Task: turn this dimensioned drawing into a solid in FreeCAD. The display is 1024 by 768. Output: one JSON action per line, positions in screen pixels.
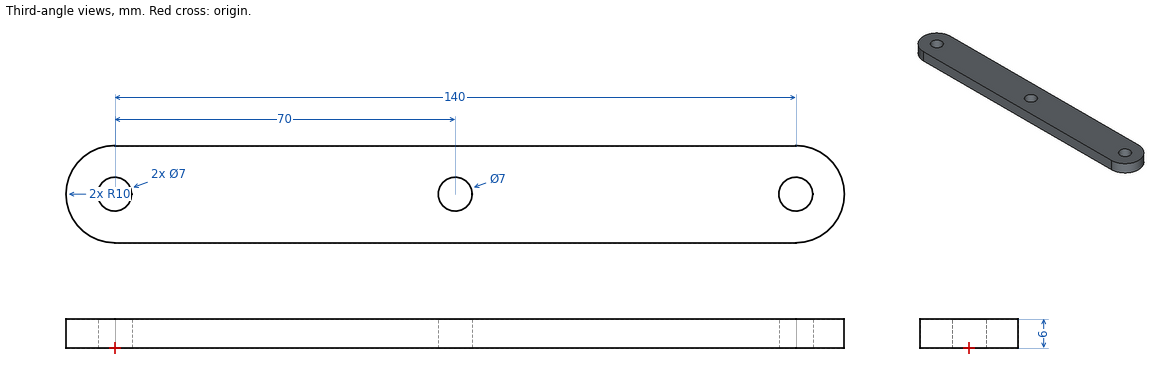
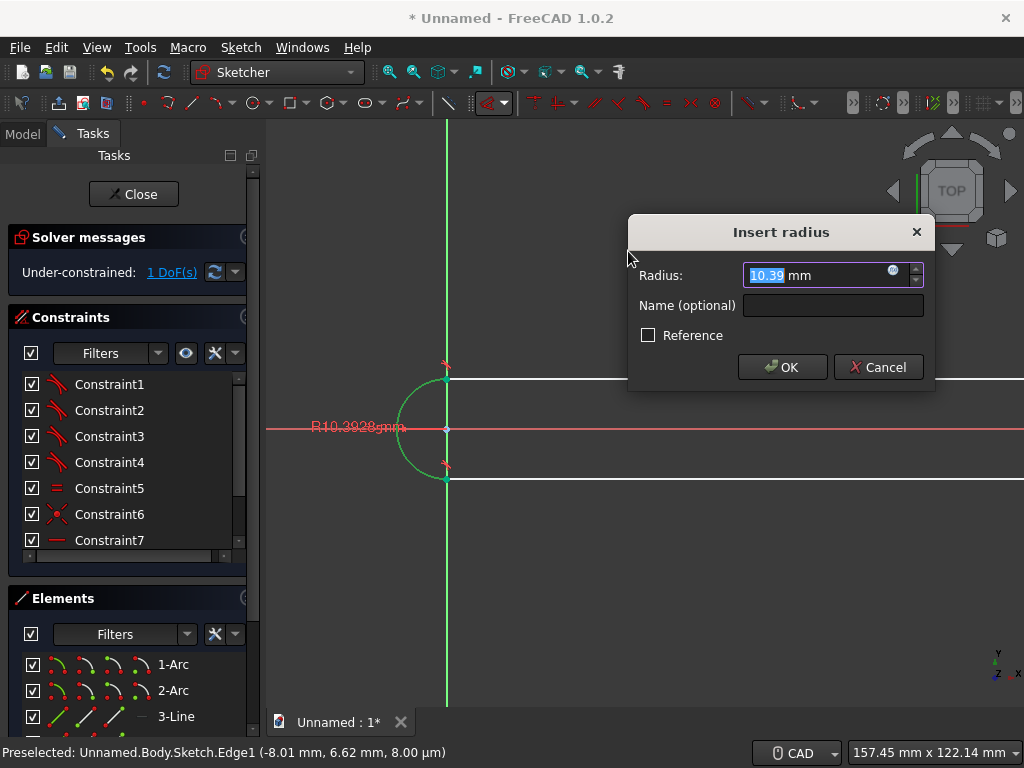
{"action": "type", "text": "10"}
{"action": "key", "text": "Return"}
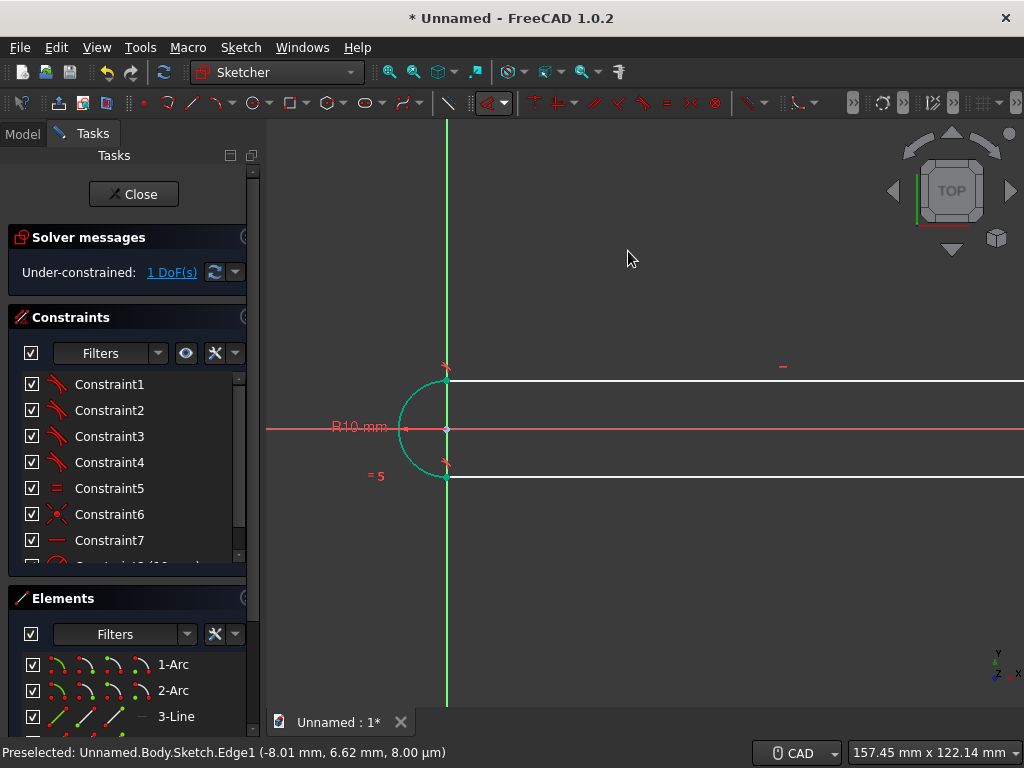
{"action": "left_click", "coordinate": [649, 381]}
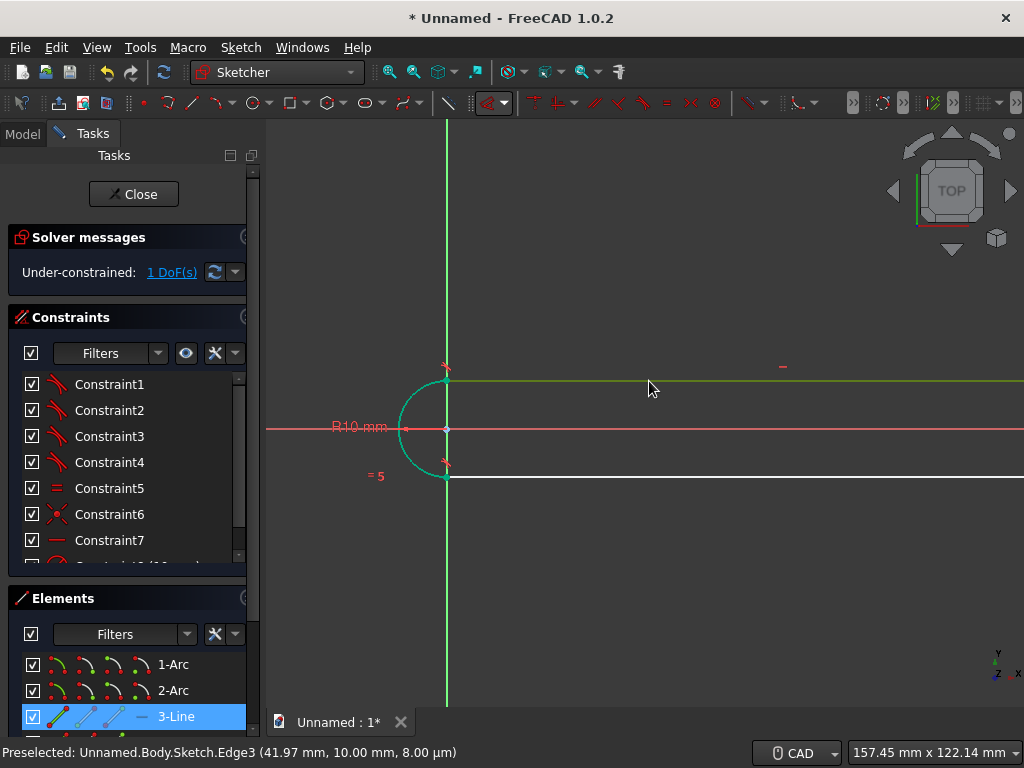
{"action": "key", "text": "l"}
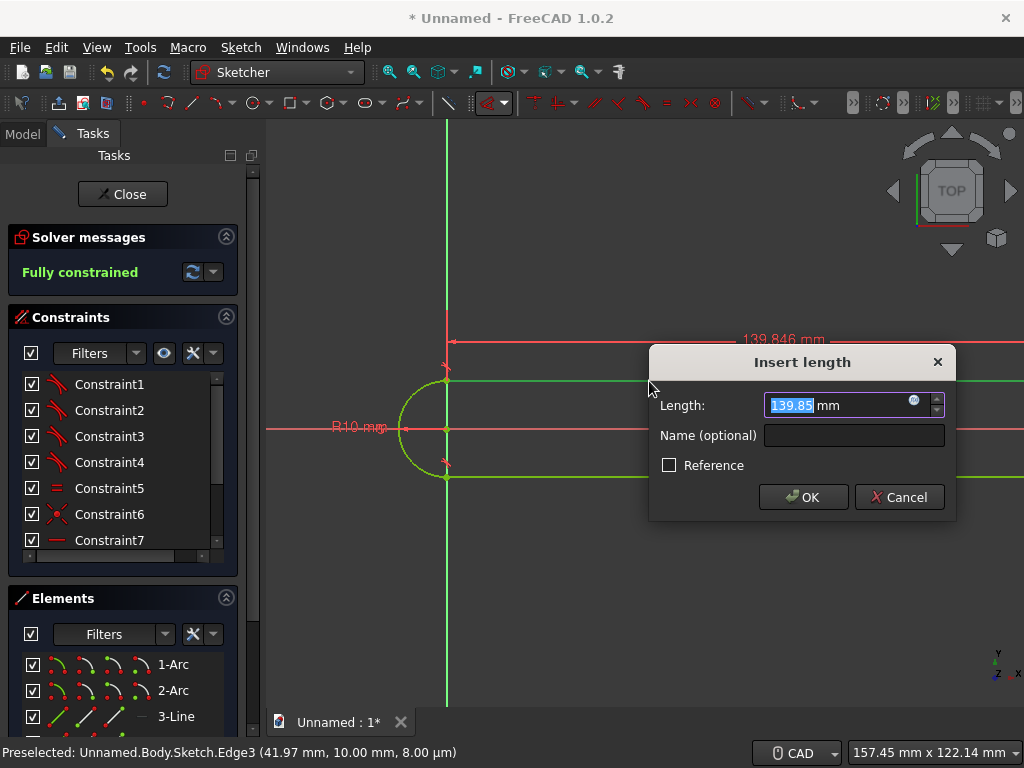
{"action": "type", "text": "140"}
{"action": "key", "text": "Return"}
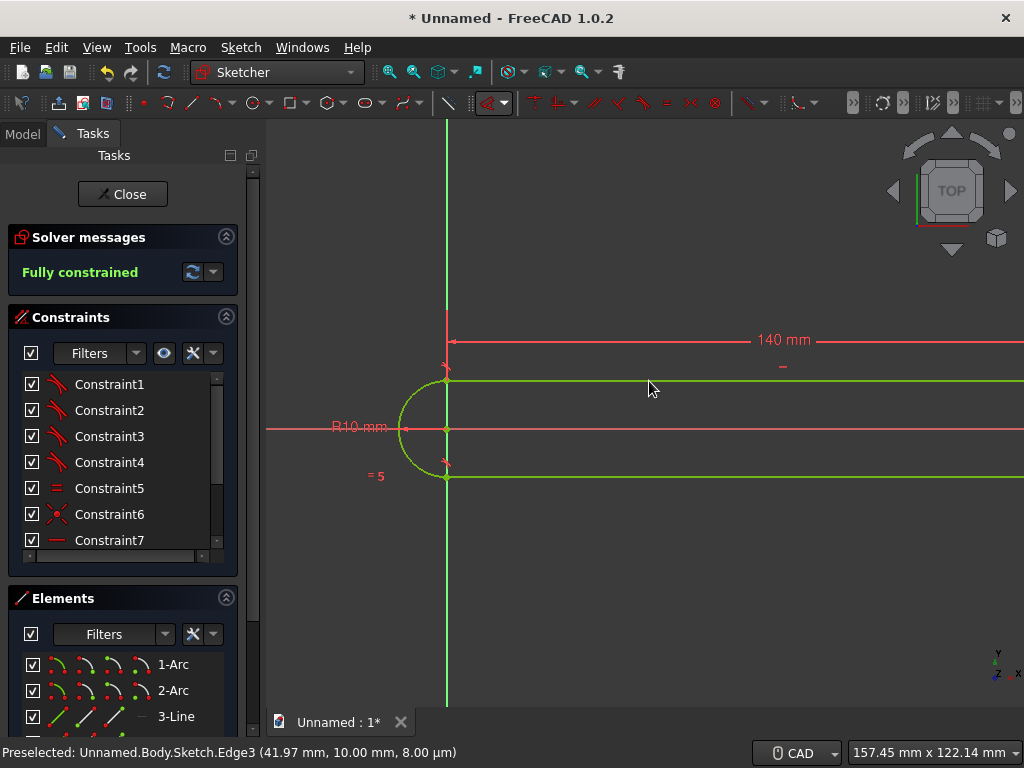
{"action": "left_click", "coordinate": [123, 194]}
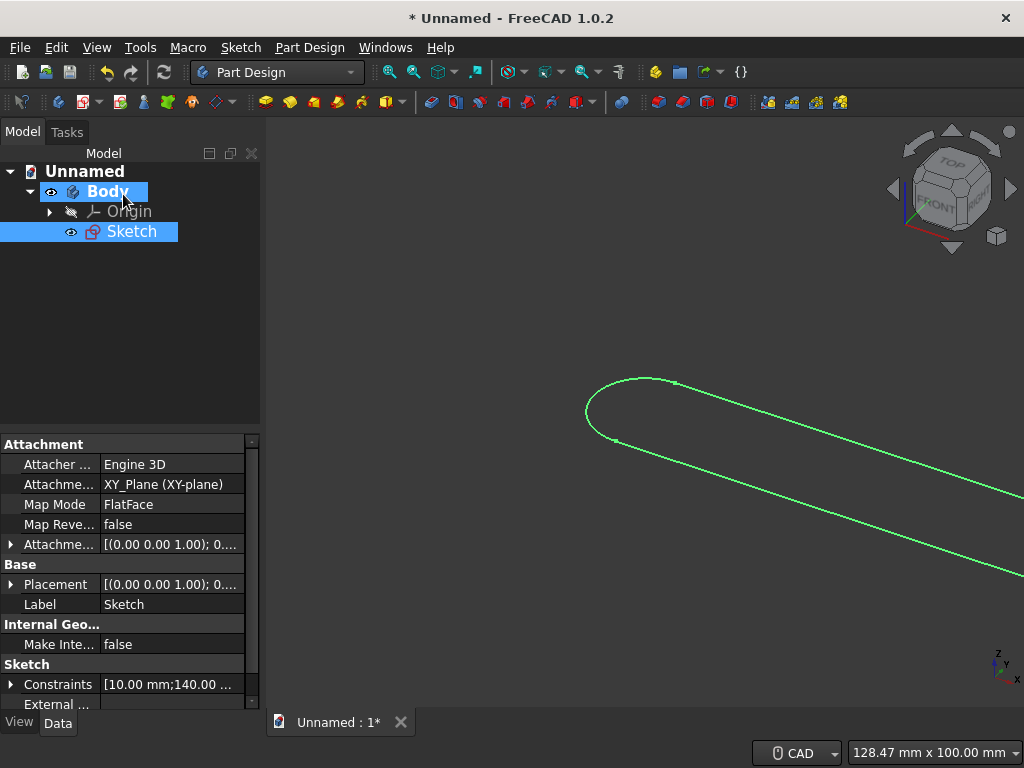
{"action": "left_click", "coordinate": [266, 102]}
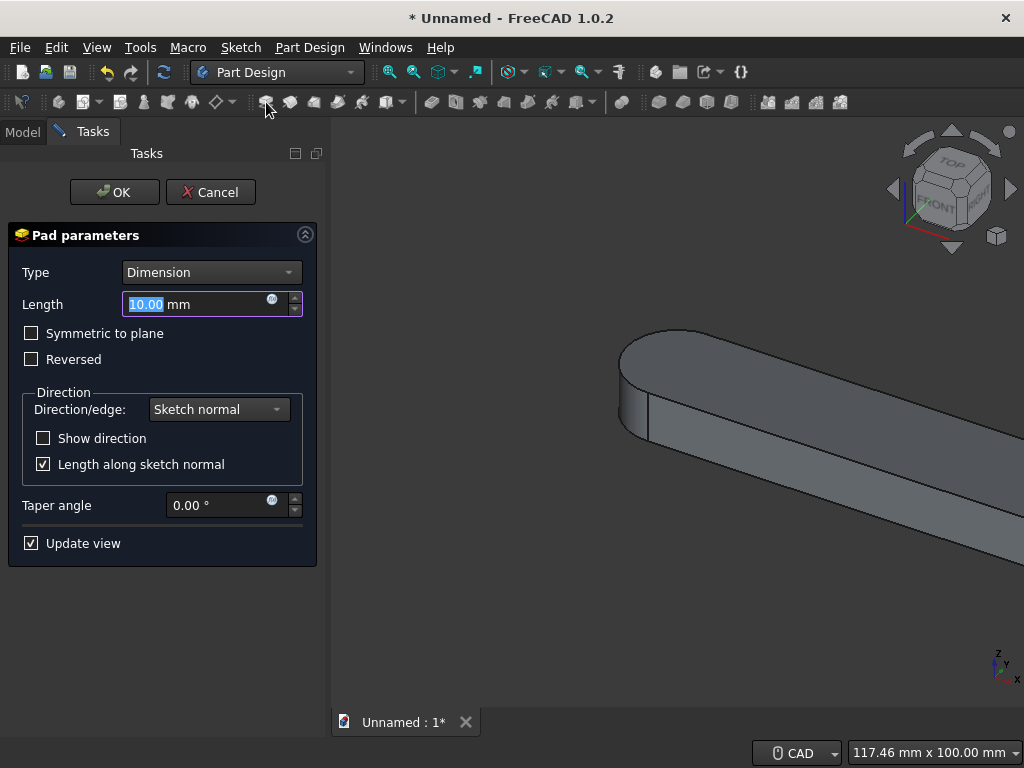
{"action": "type", "text": "6"}
{"action": "key", "text": "Tab"}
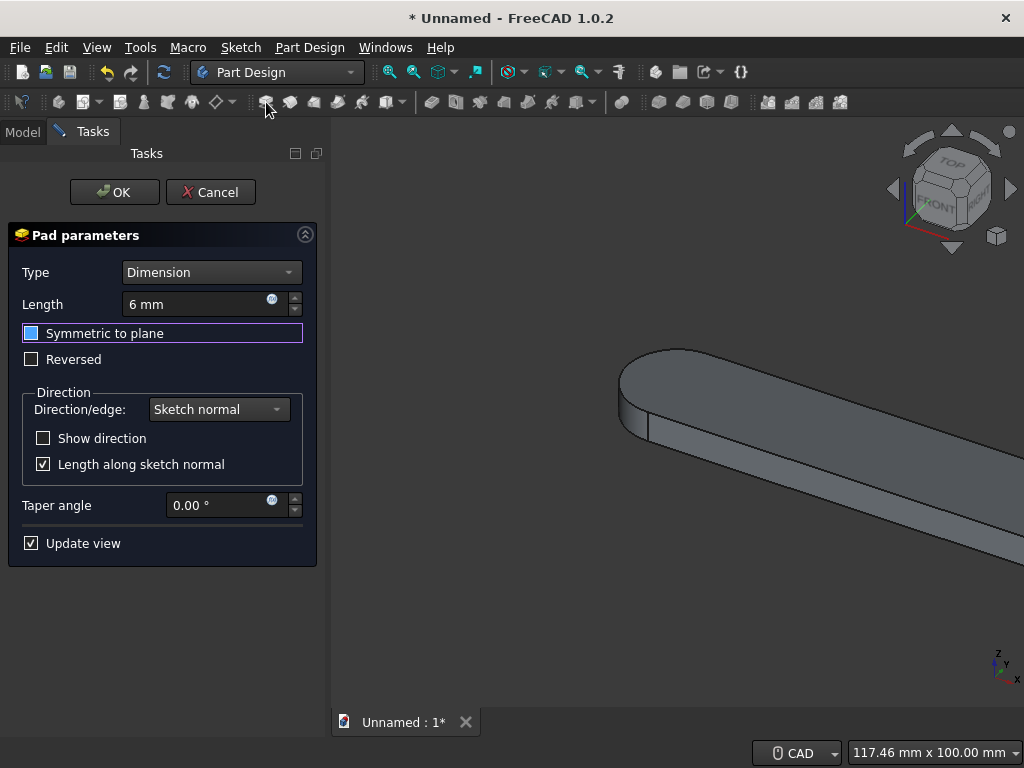
{"action": "left_click", "coordinate": [115, 192]}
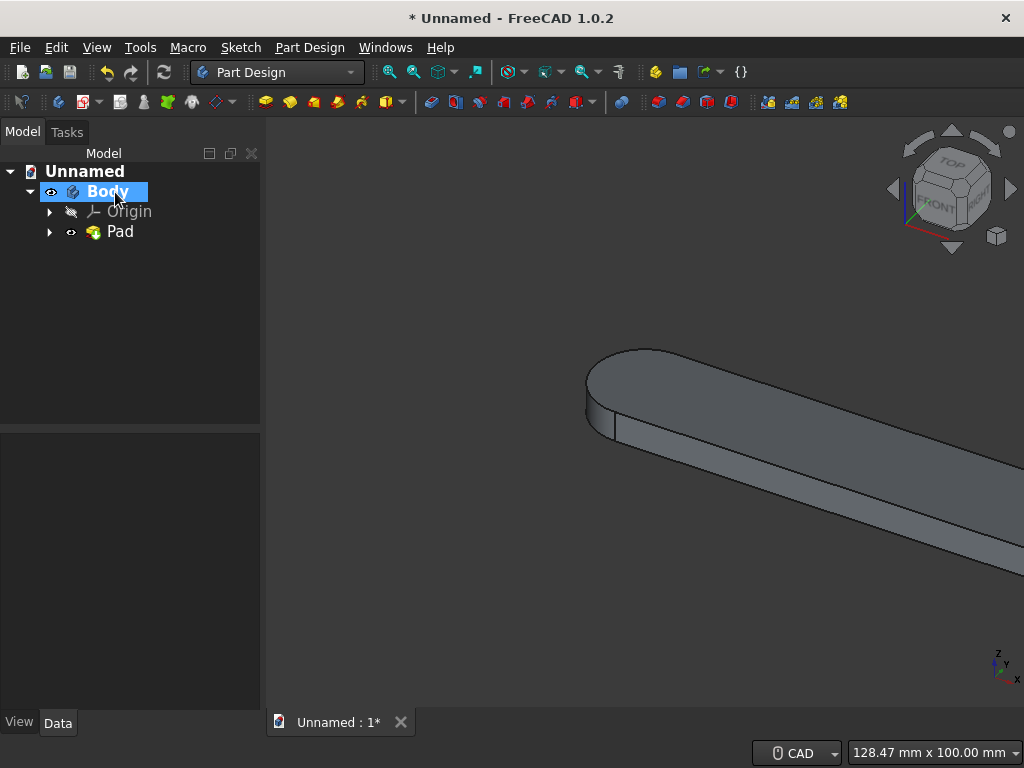
{"action": "left_click", "coordinate": [390, 72]}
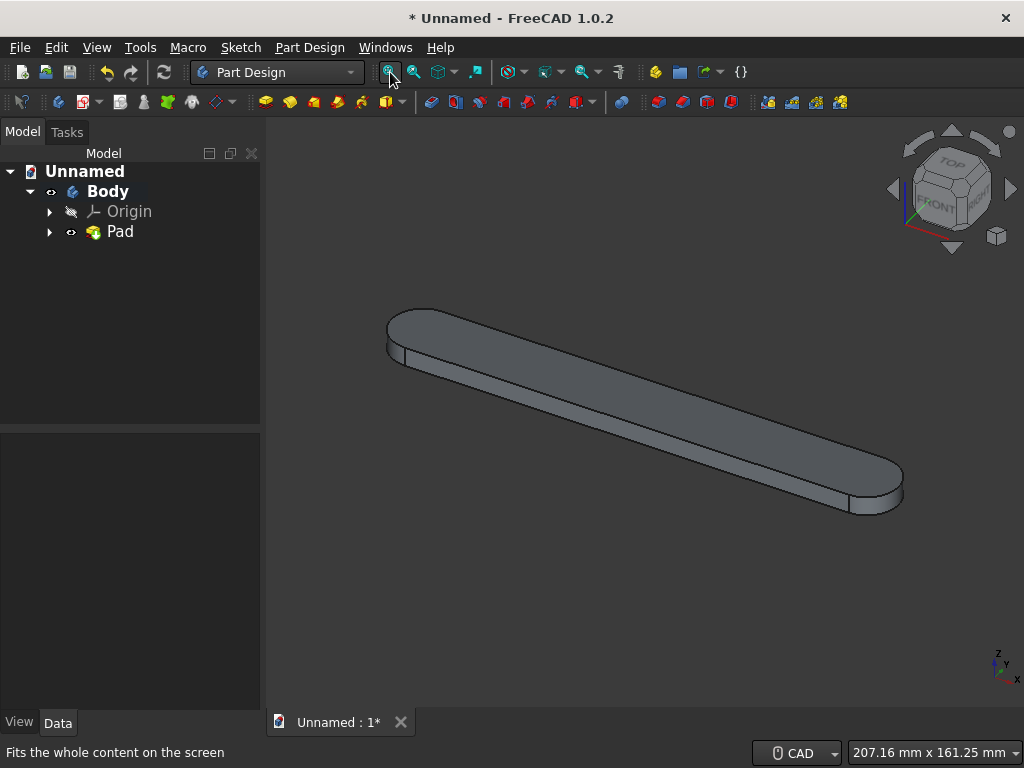
{"action": "left_click", "coordinate": [862, 474]}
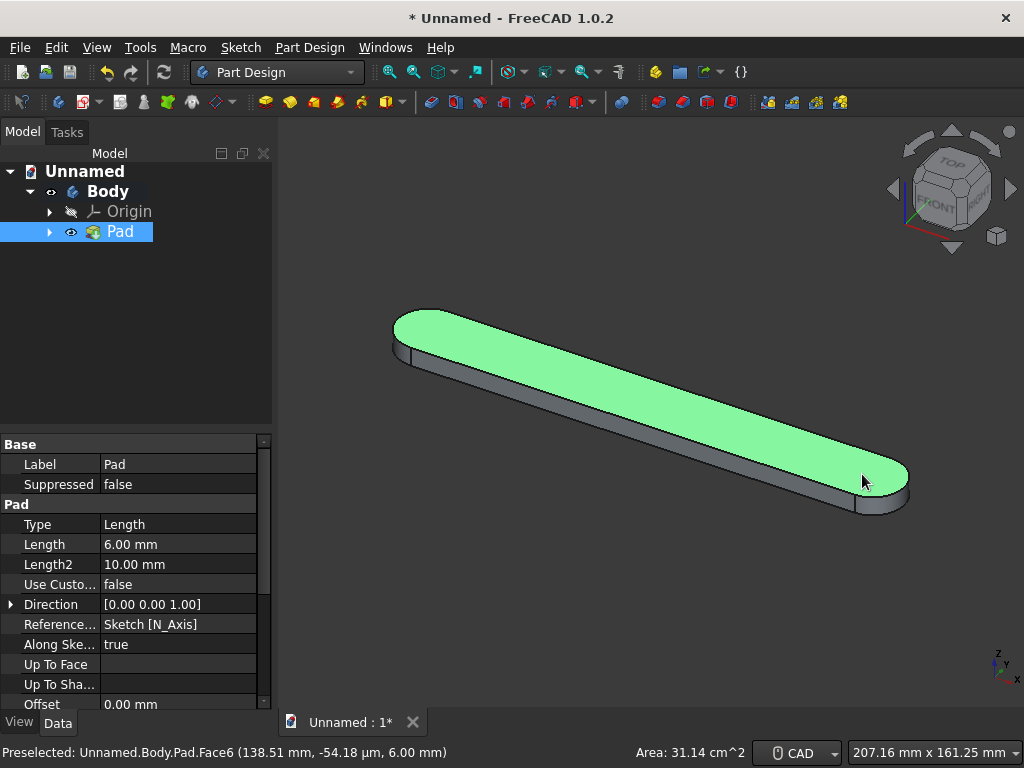
{"action": "left_click", "coordinate": [84, 102]}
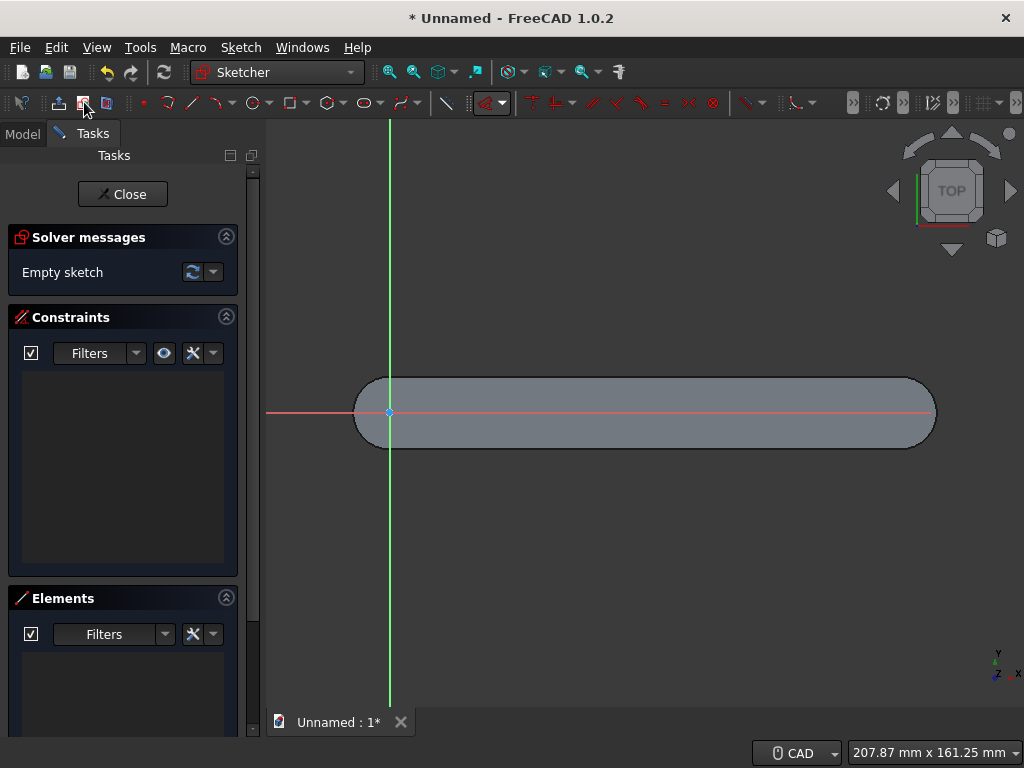
{"action": "scroll", "coordinate": [294, 413], "scroll_direction": "down", "scroll_amount": 1}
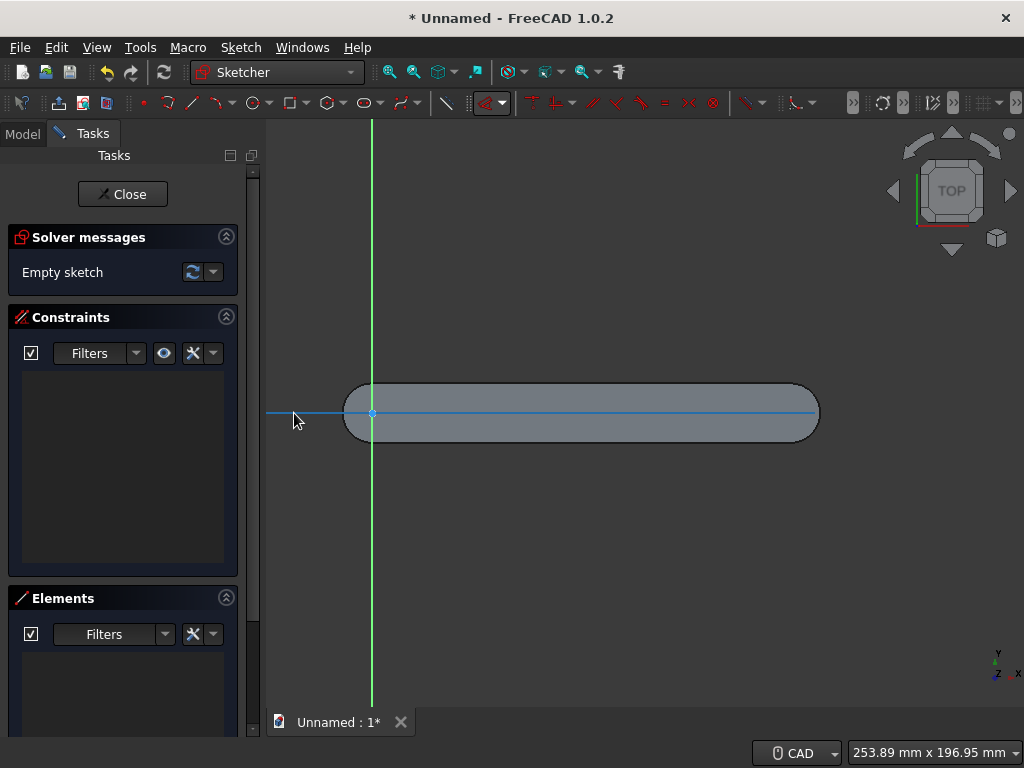
{"action": "left_click", "coordinate": [254, 104]}